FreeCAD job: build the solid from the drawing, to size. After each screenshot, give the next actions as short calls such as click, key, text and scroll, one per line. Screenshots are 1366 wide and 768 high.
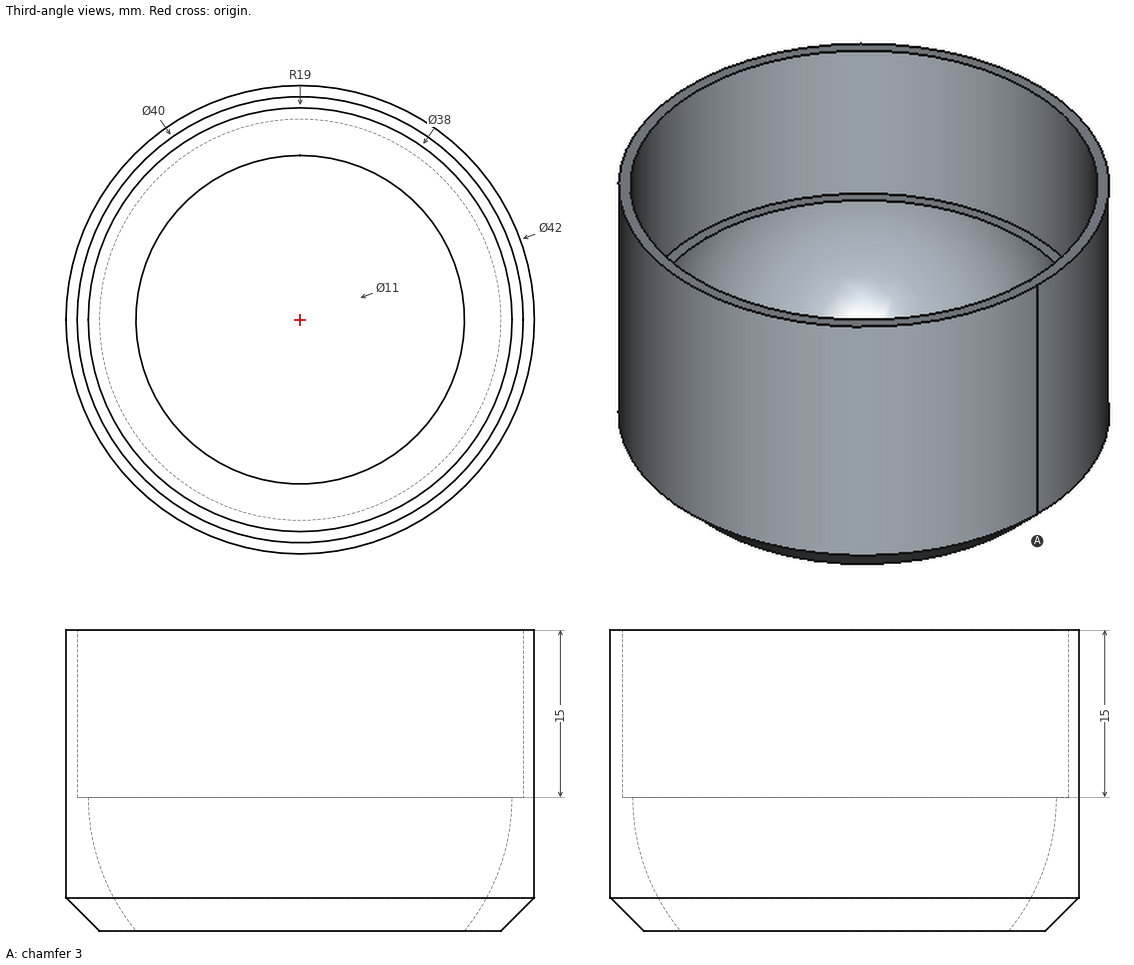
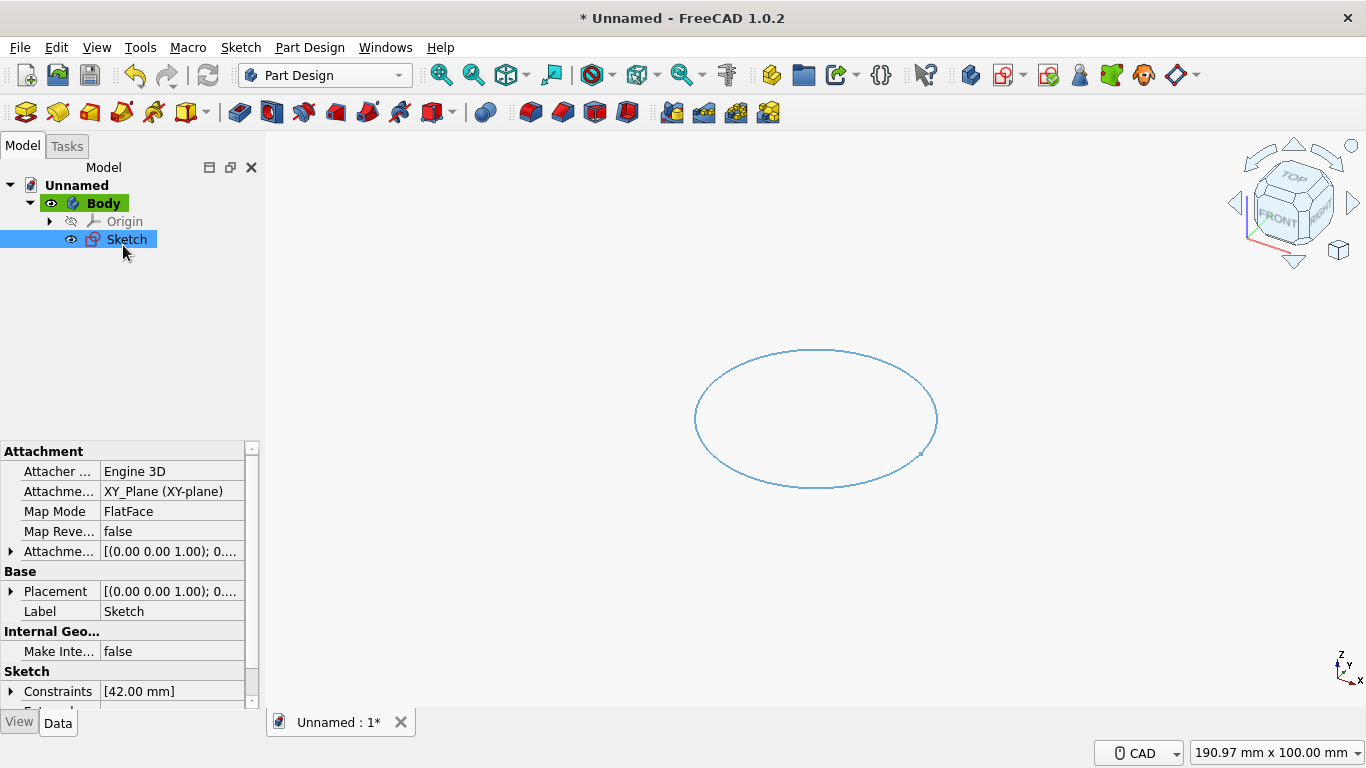
click(26, 112)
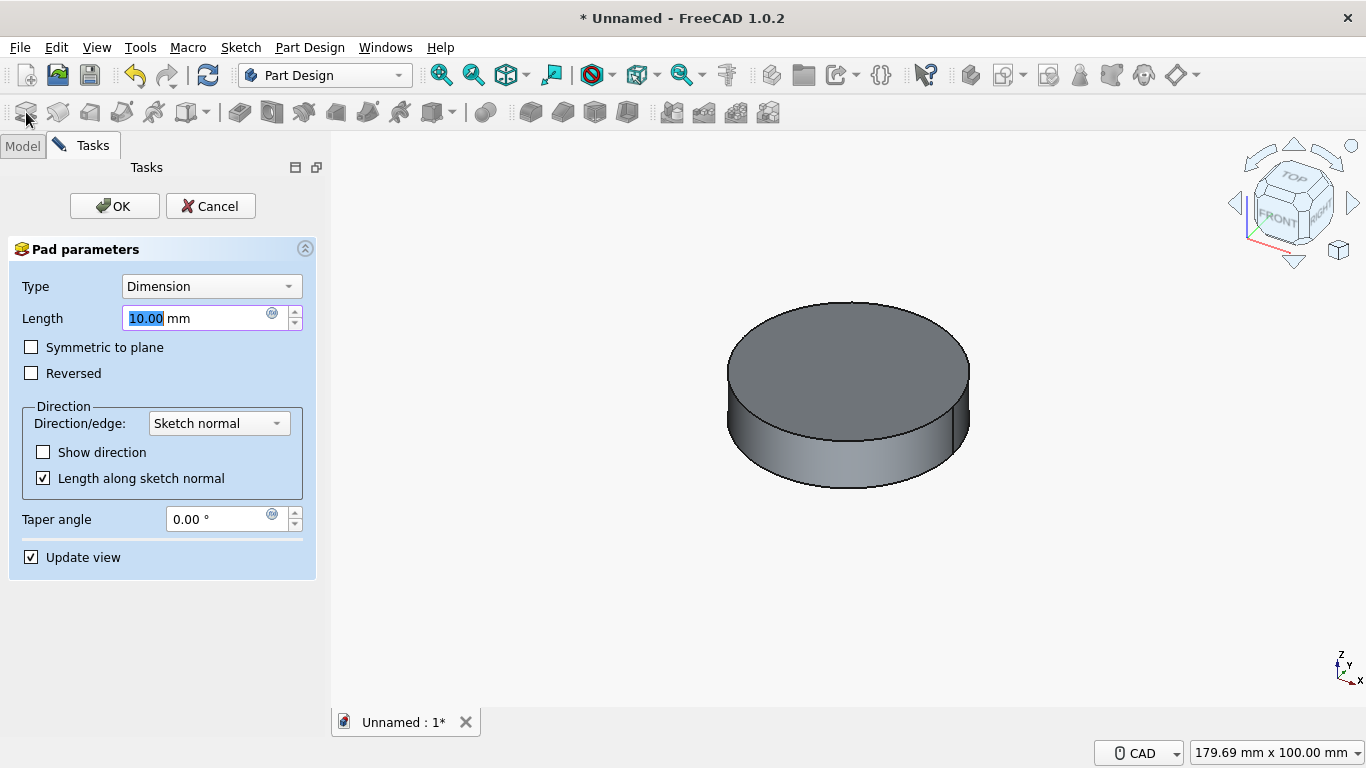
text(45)
key(Tab)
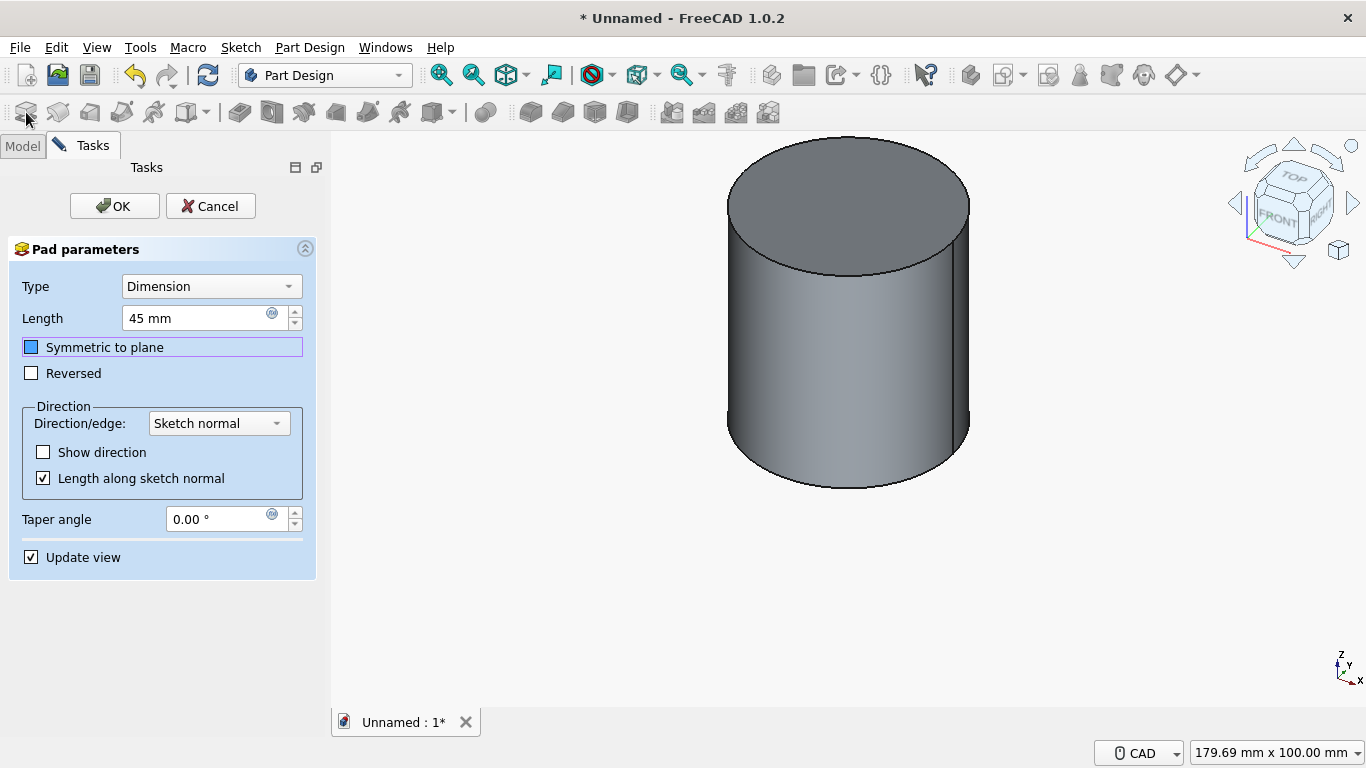
click(115, 206)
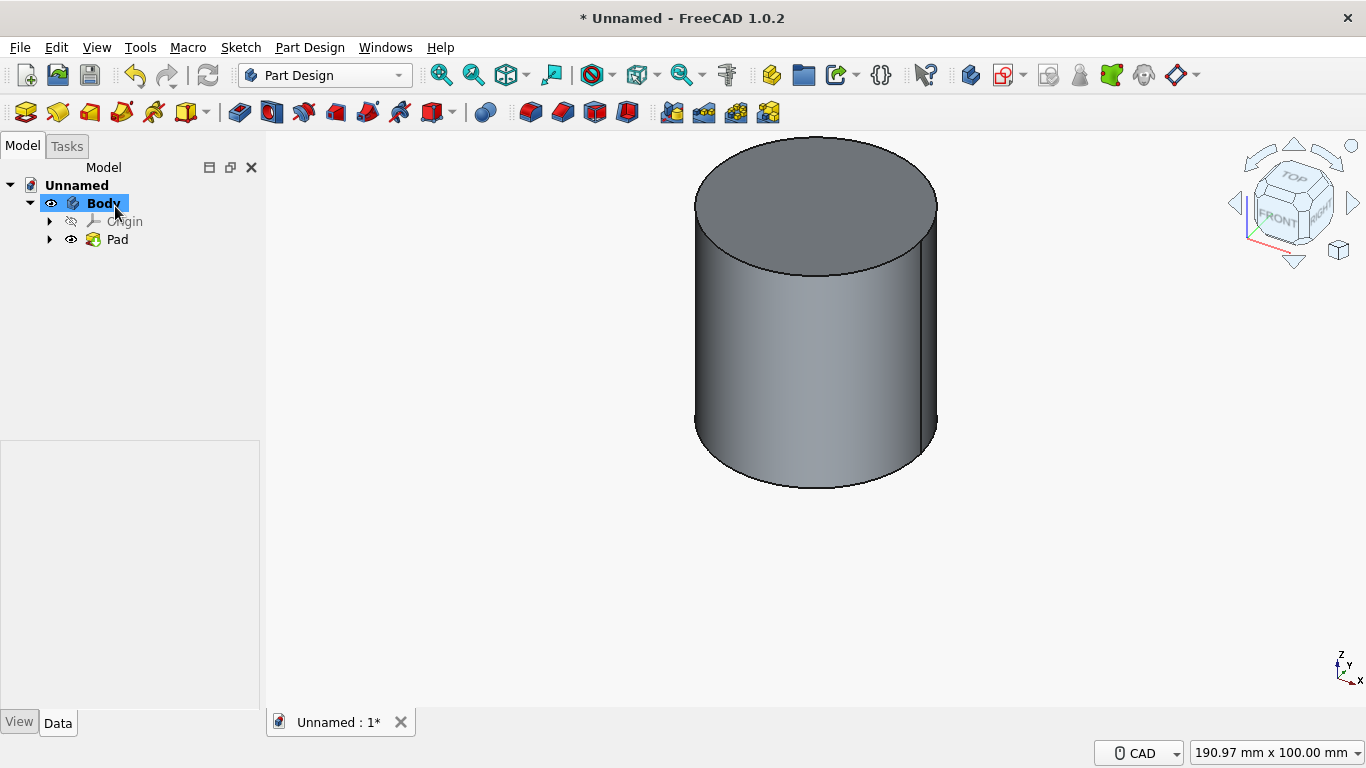
click(442, 76)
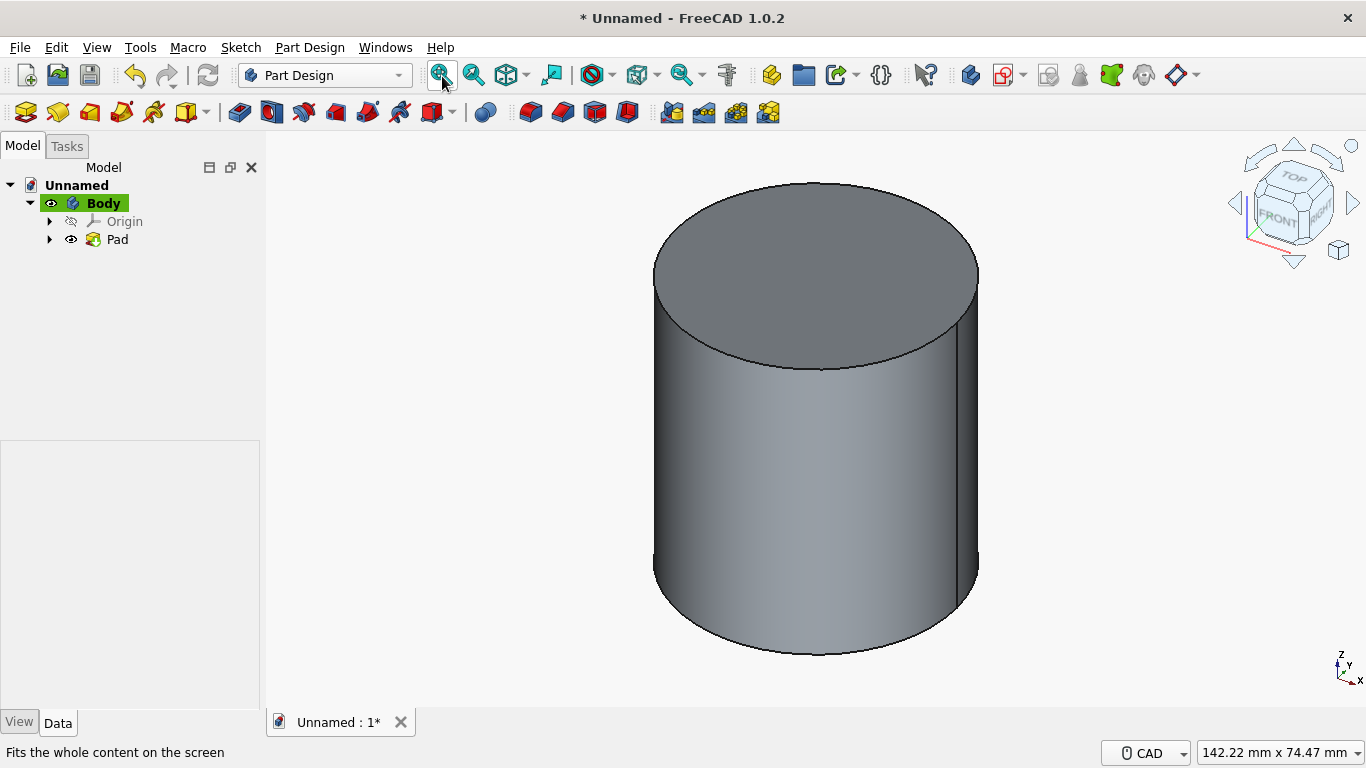
click(816, 275)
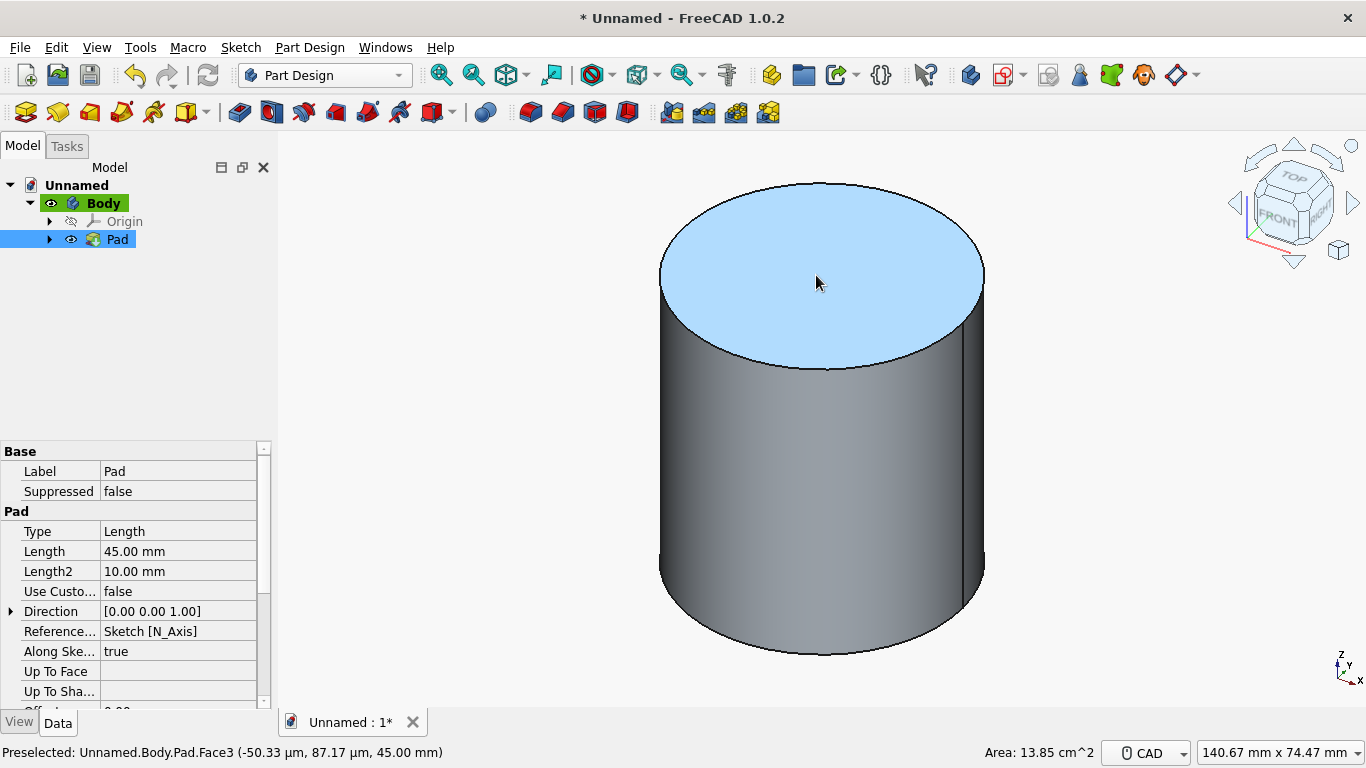
click(1004, 76)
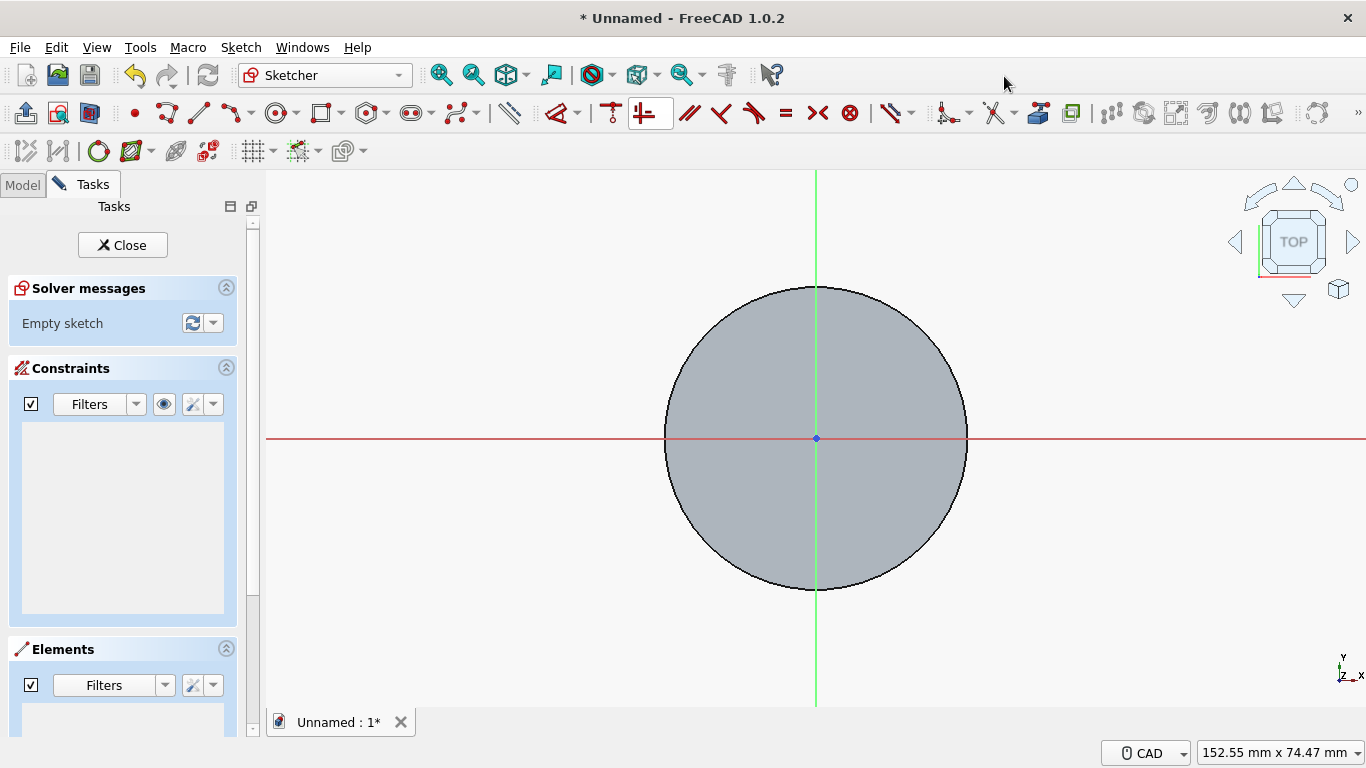
click(276, 114)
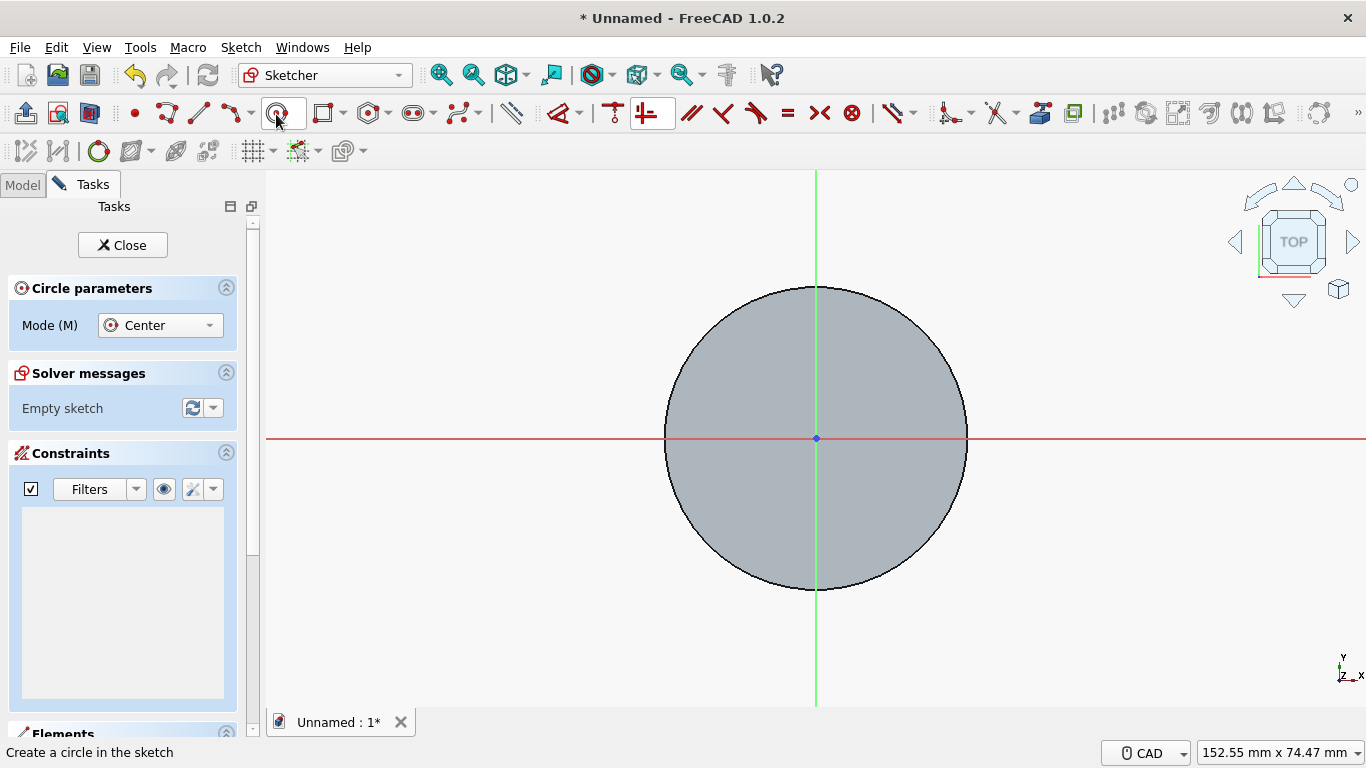
click(816, 438)
move(913, 342)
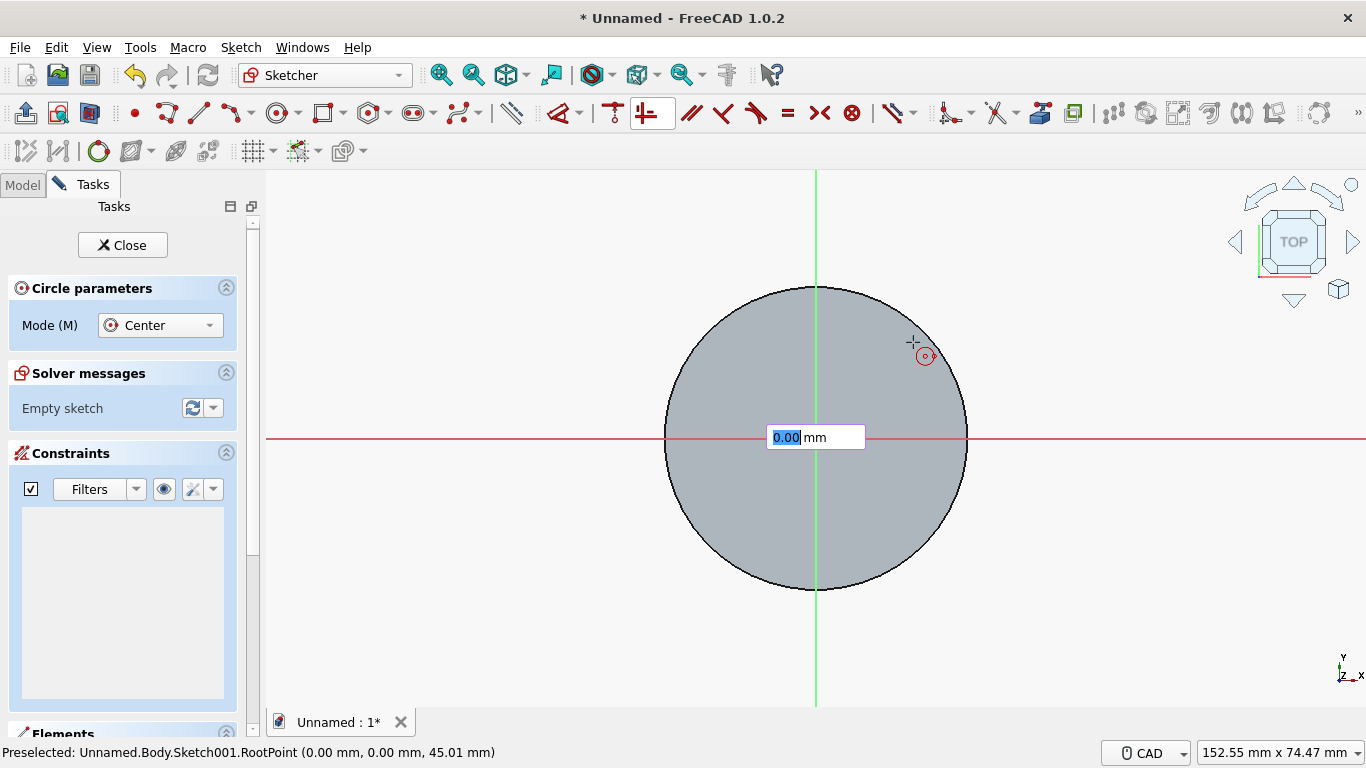
text(38)
key(Return)
key(Escape)